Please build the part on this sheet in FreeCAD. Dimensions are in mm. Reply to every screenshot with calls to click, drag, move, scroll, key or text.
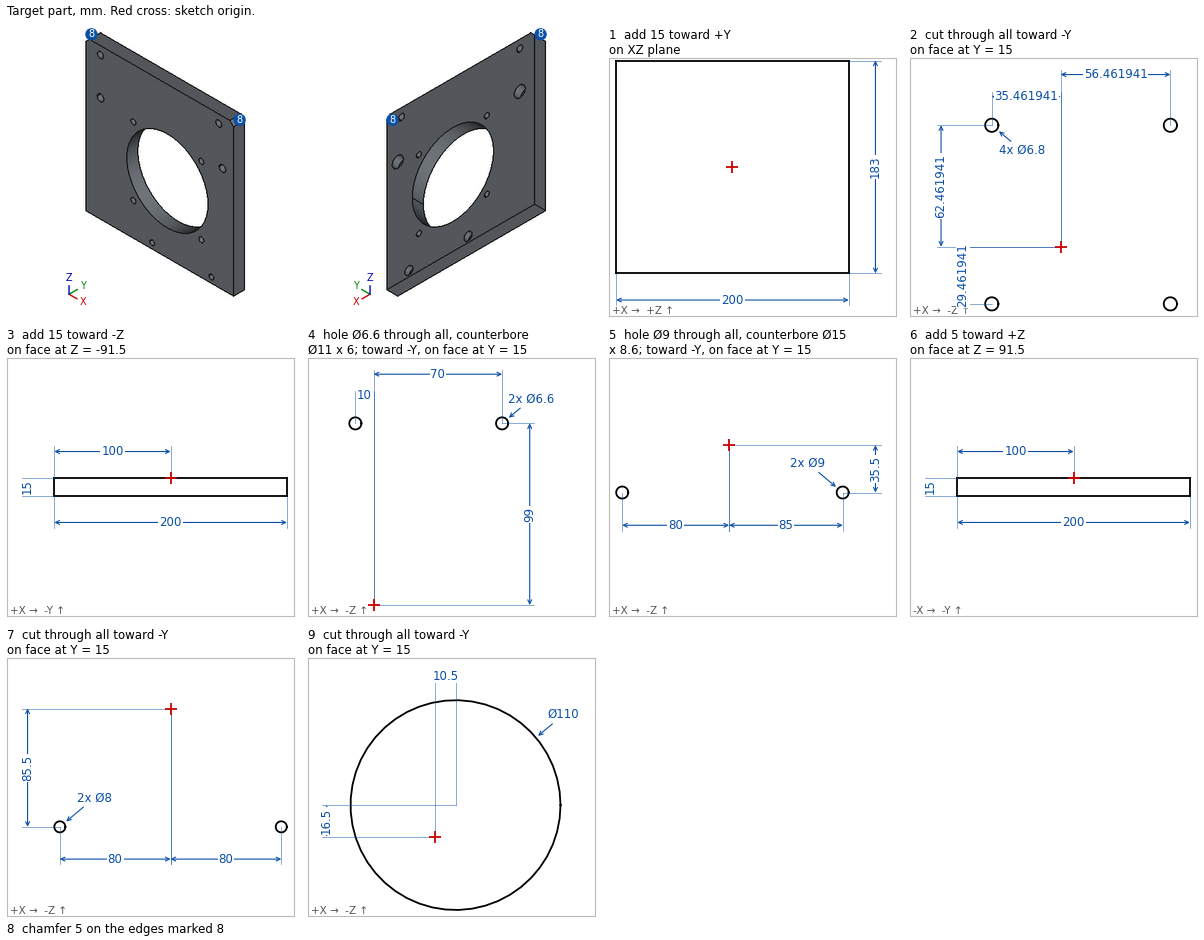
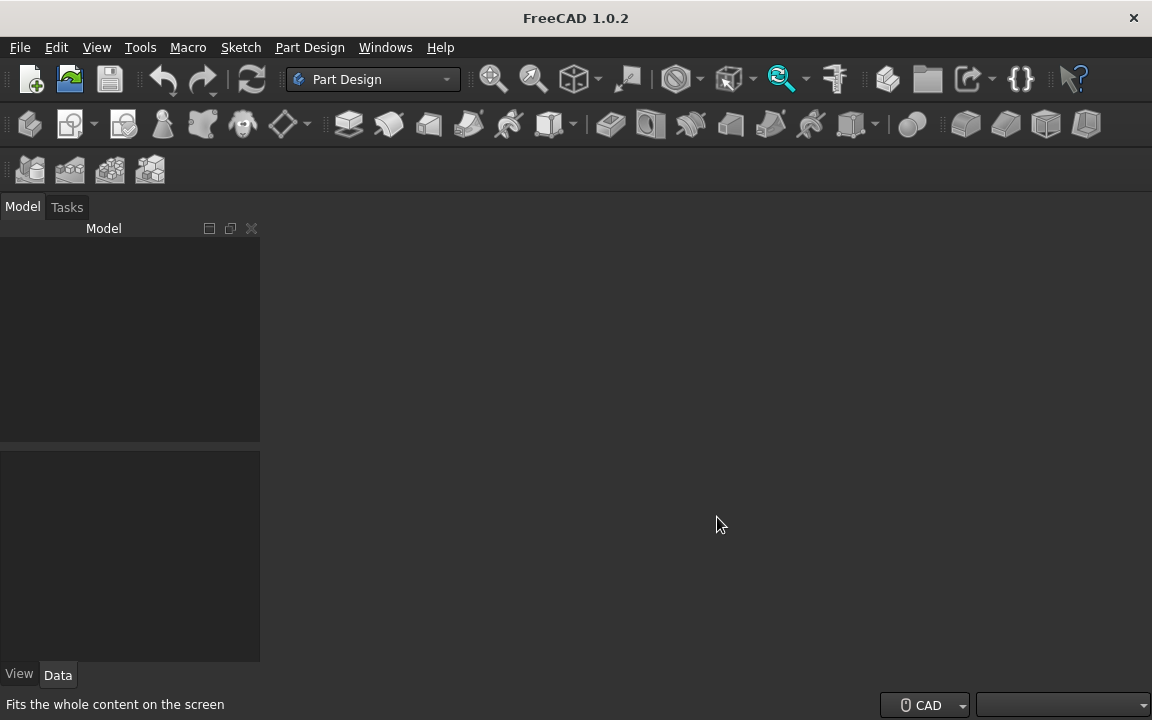
key(ctrl+n)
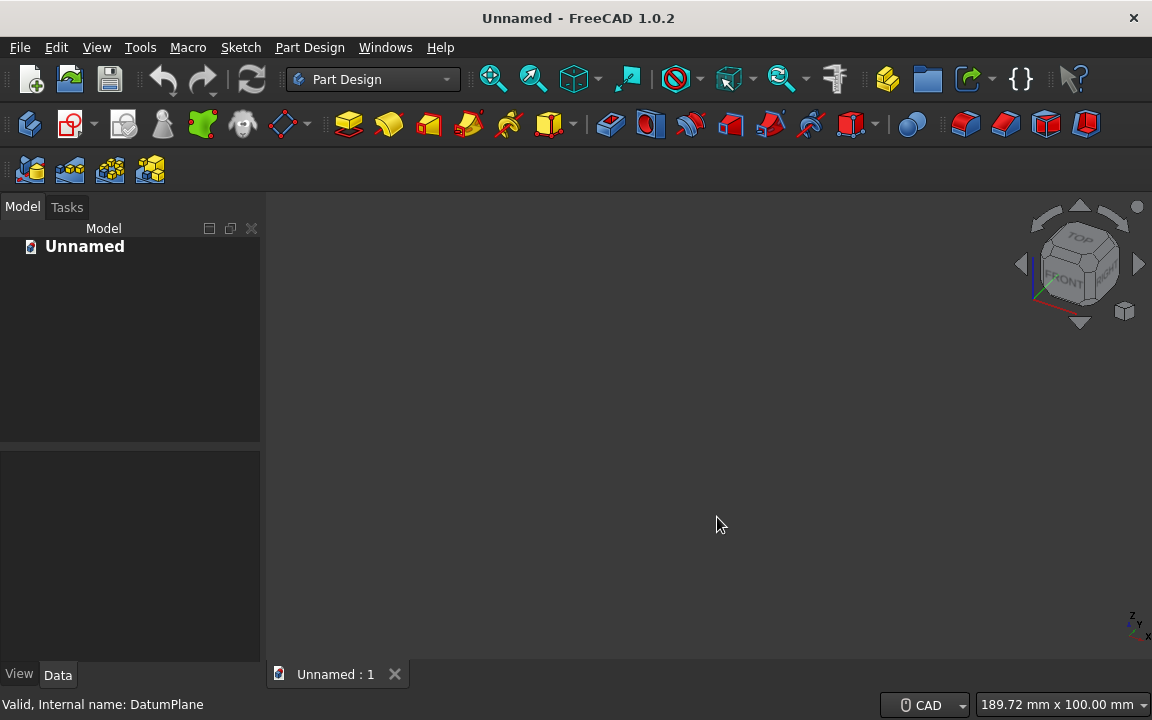
click(70, 124)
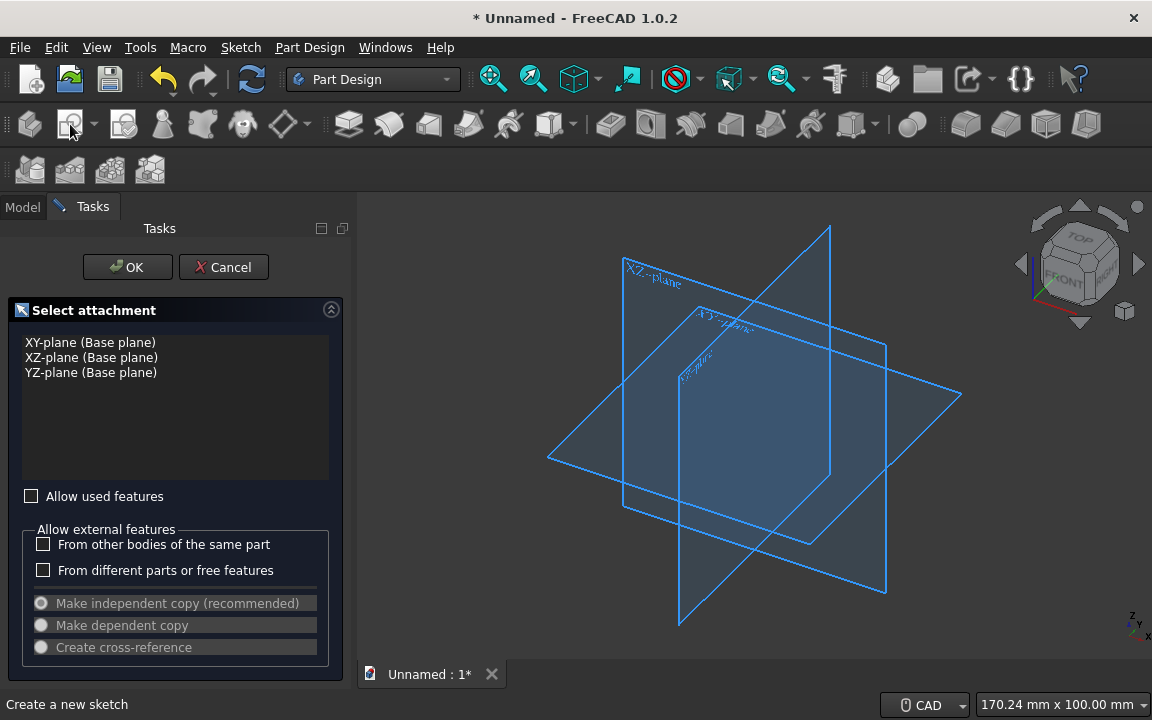
click(82, 358)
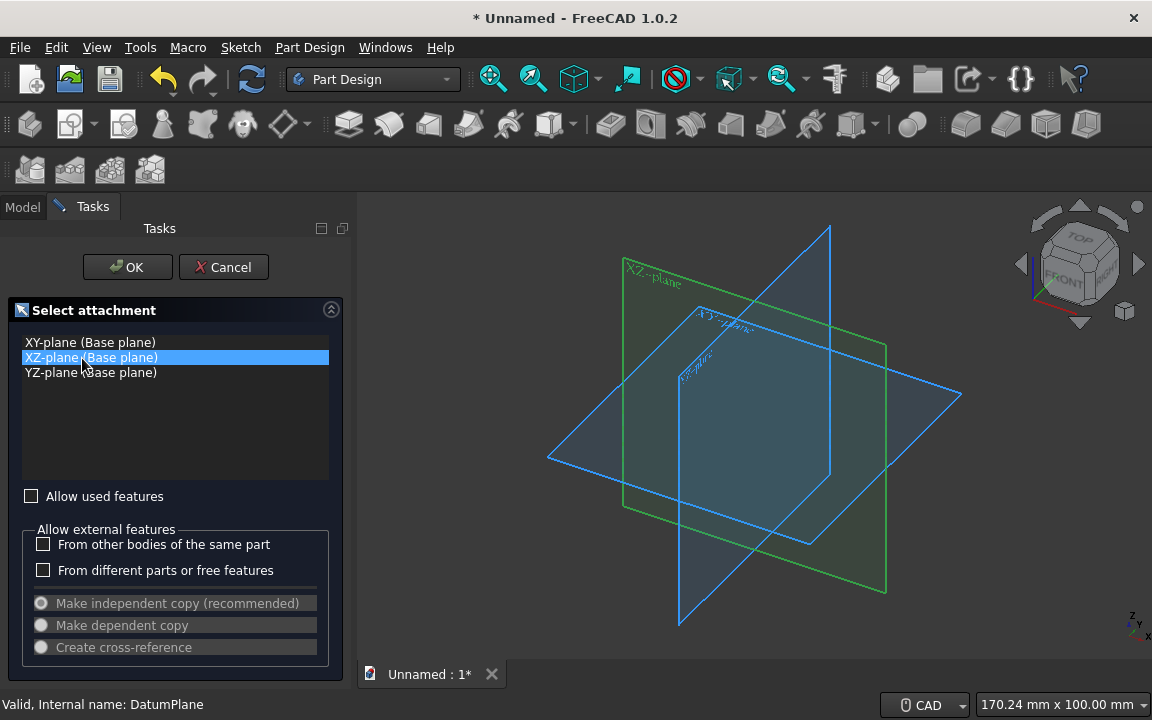
click(128, 267)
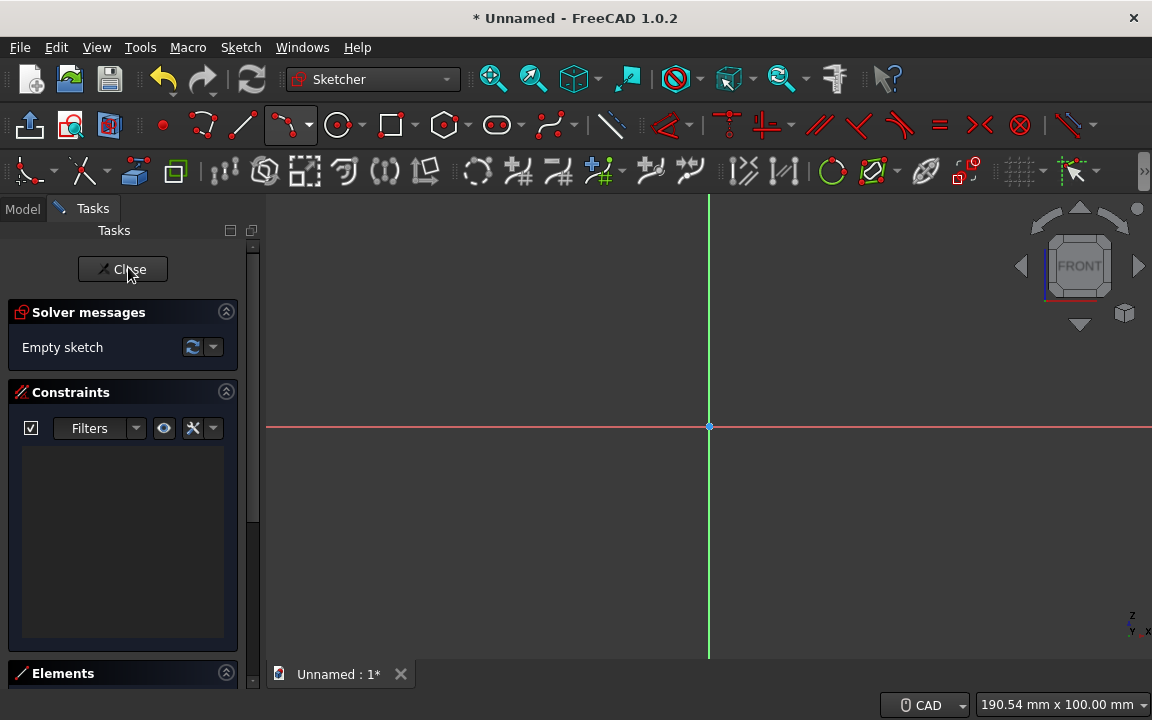
scroll(601, 427, down, 5)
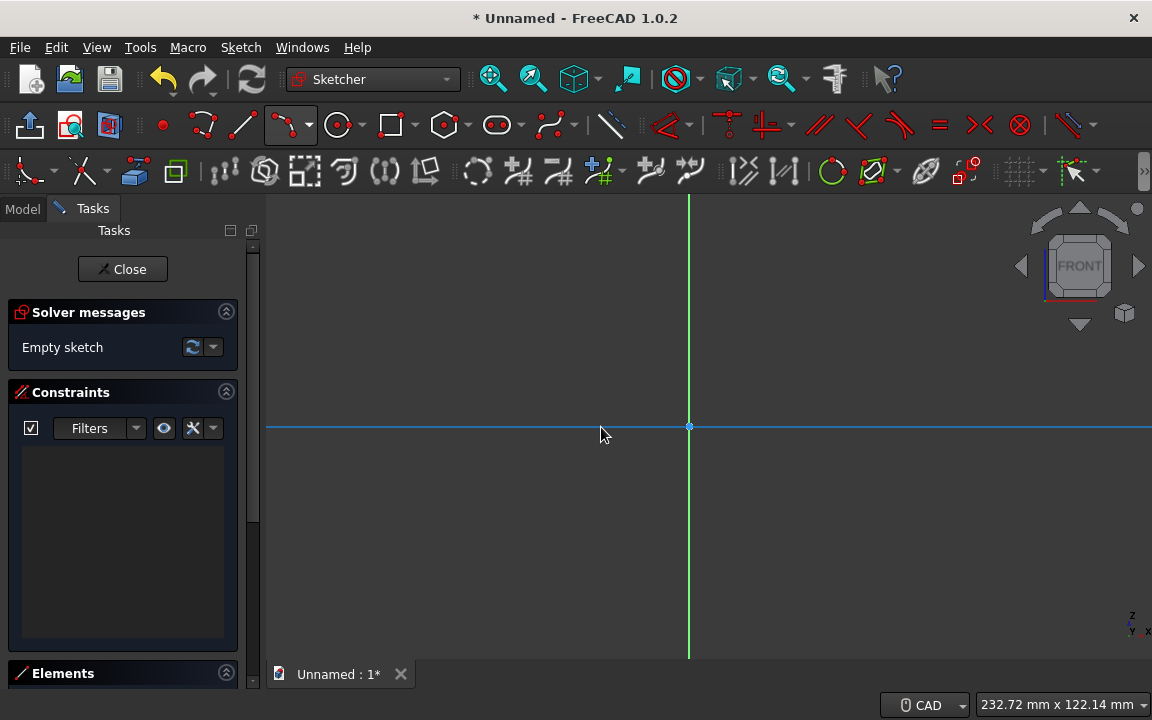
click(418, 126)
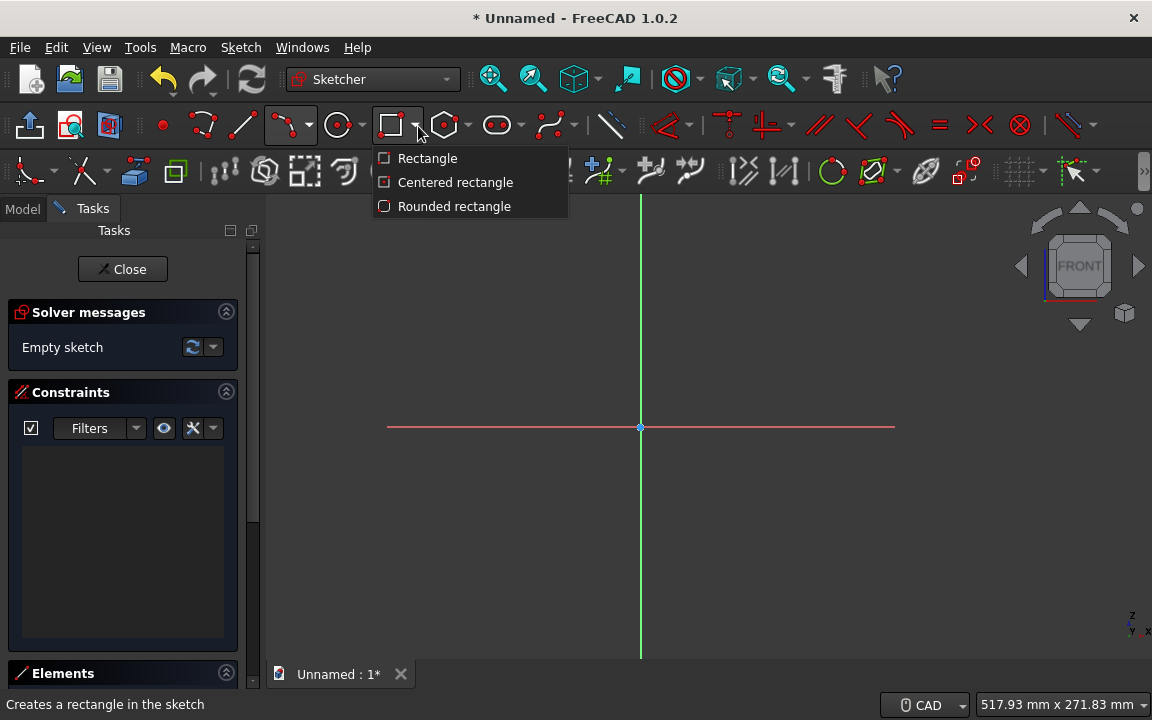
click(470, 182)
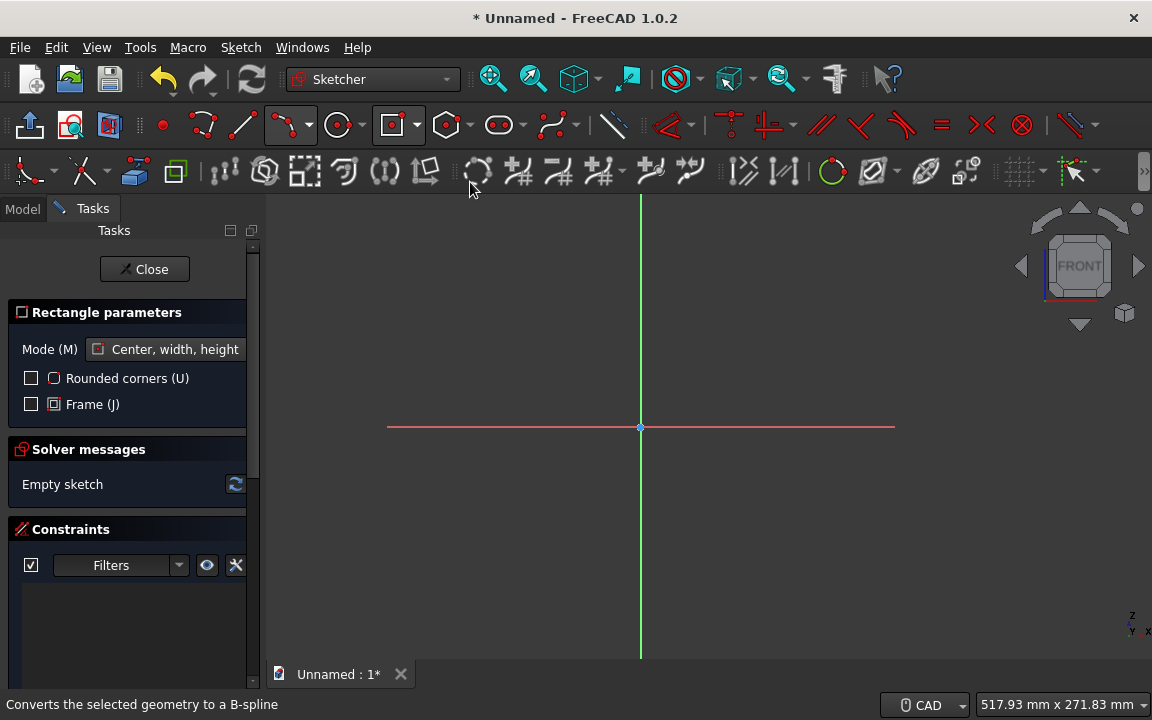
click(641, 427)
click(812, 271)
key(Escape)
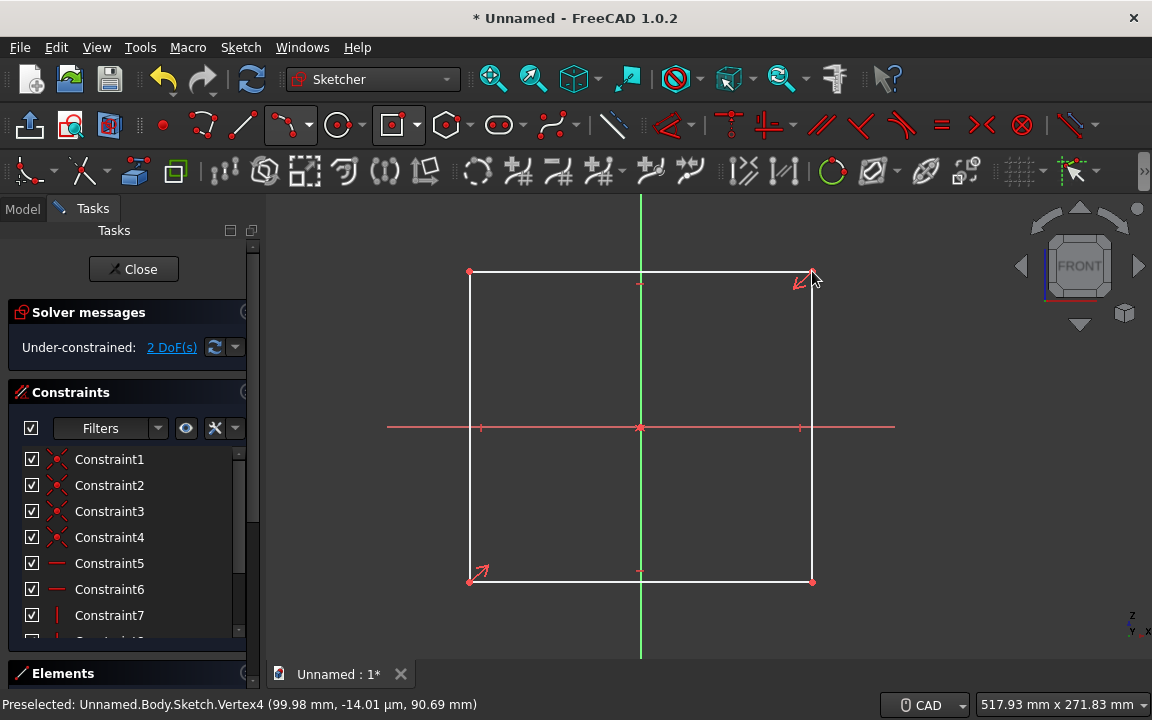
key(d)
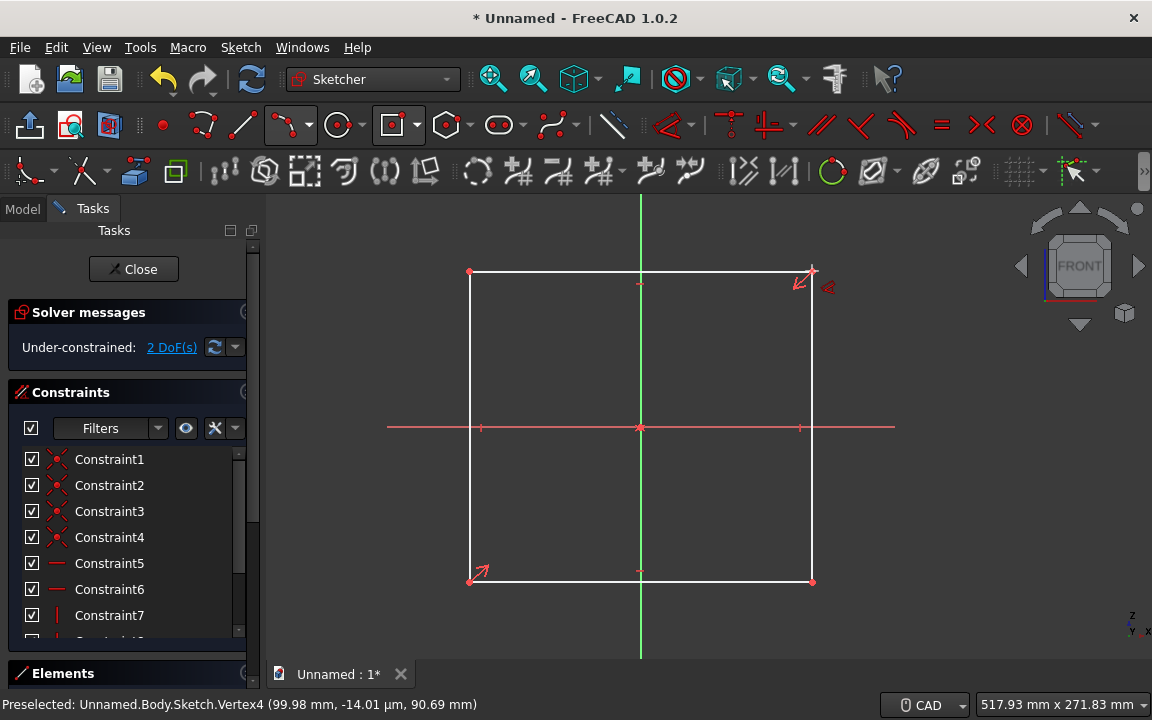
click(573, 582)
click(562, 616)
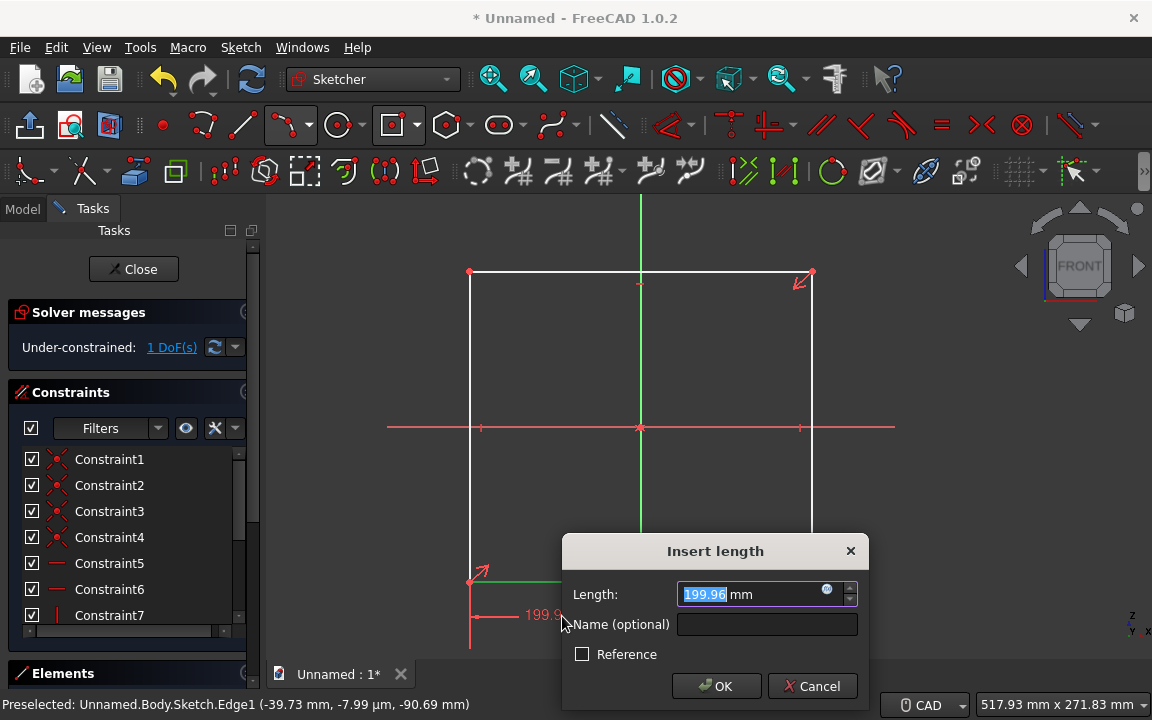
text(200)
key(Return)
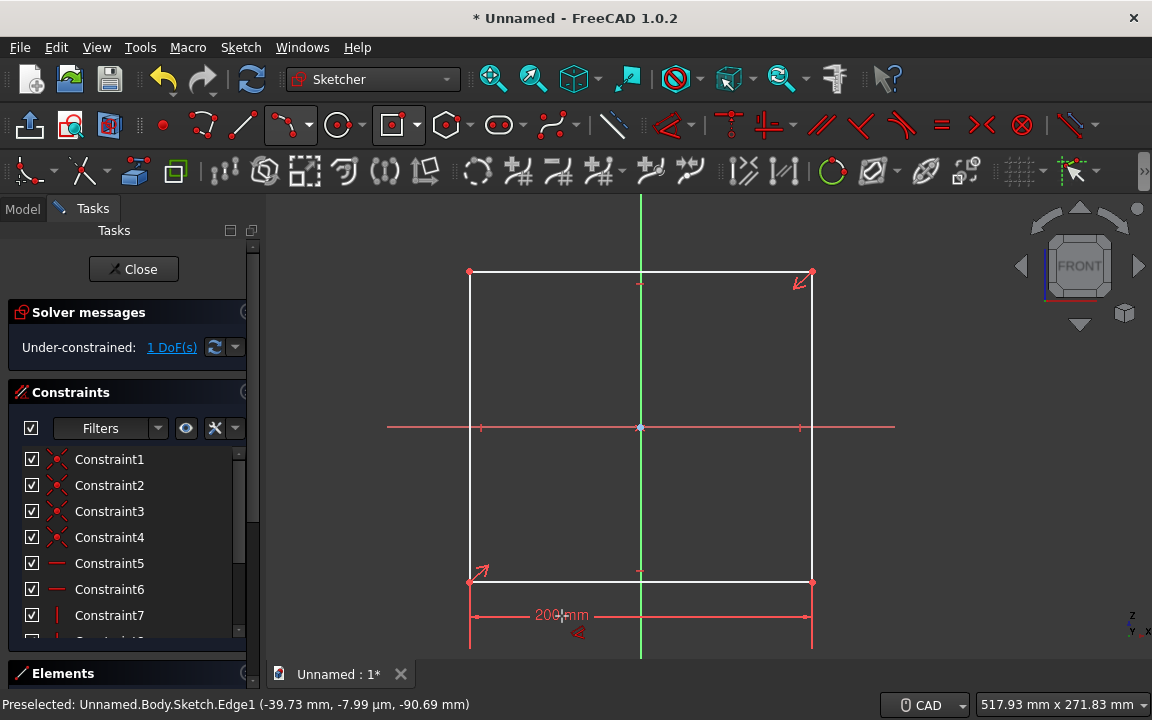
click(812, 489)
click(846, 356)